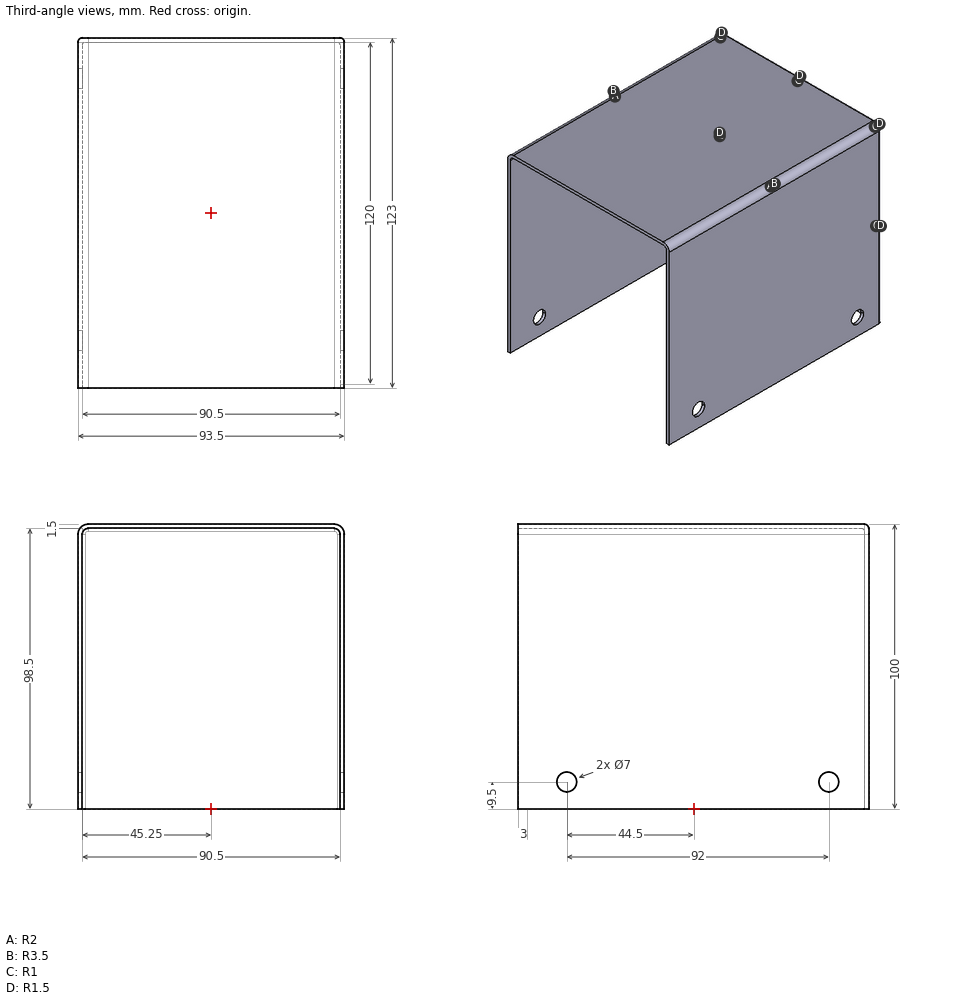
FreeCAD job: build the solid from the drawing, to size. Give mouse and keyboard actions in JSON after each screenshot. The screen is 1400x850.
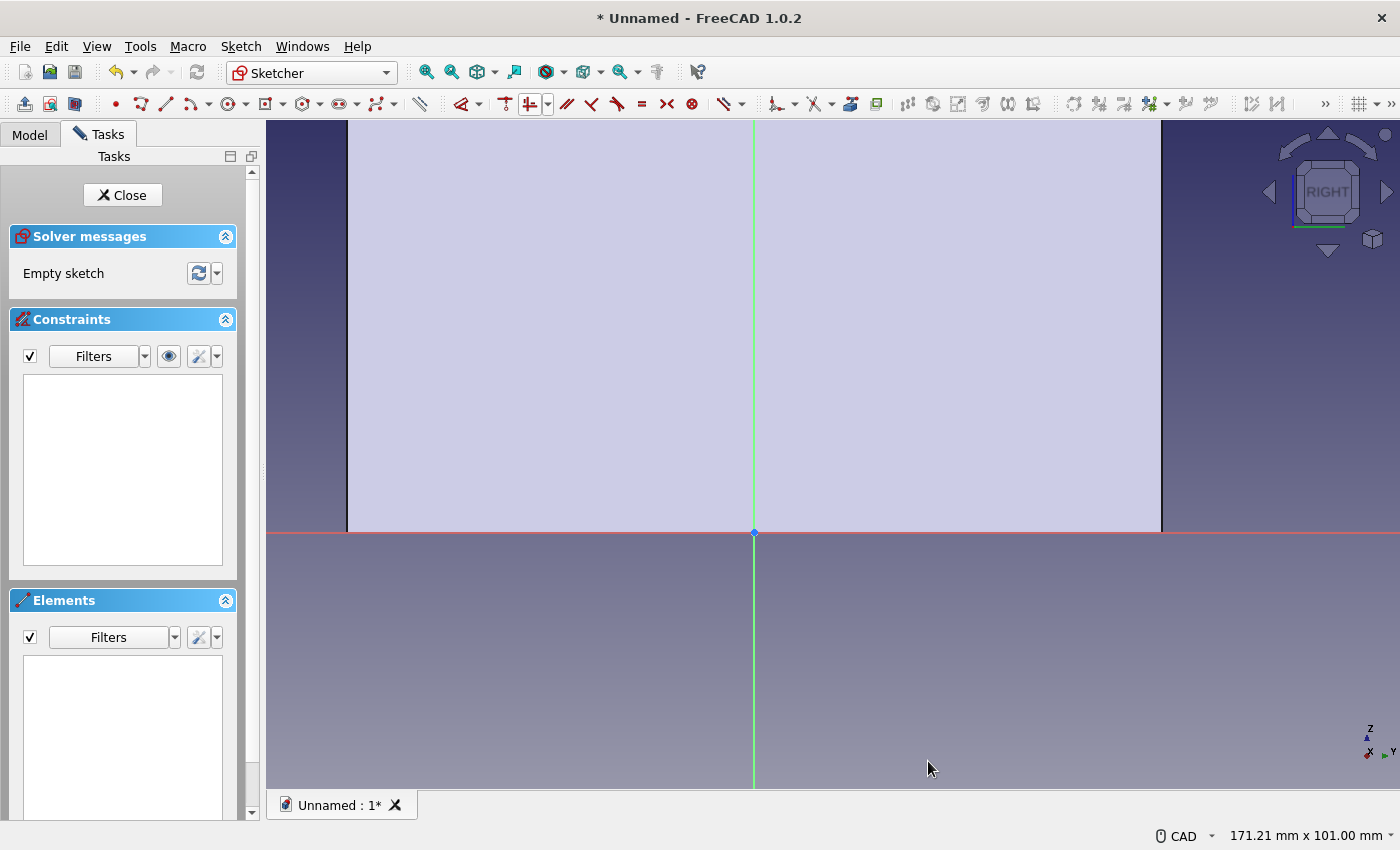
{"action": "left_click", "coordinate": [228, 104]}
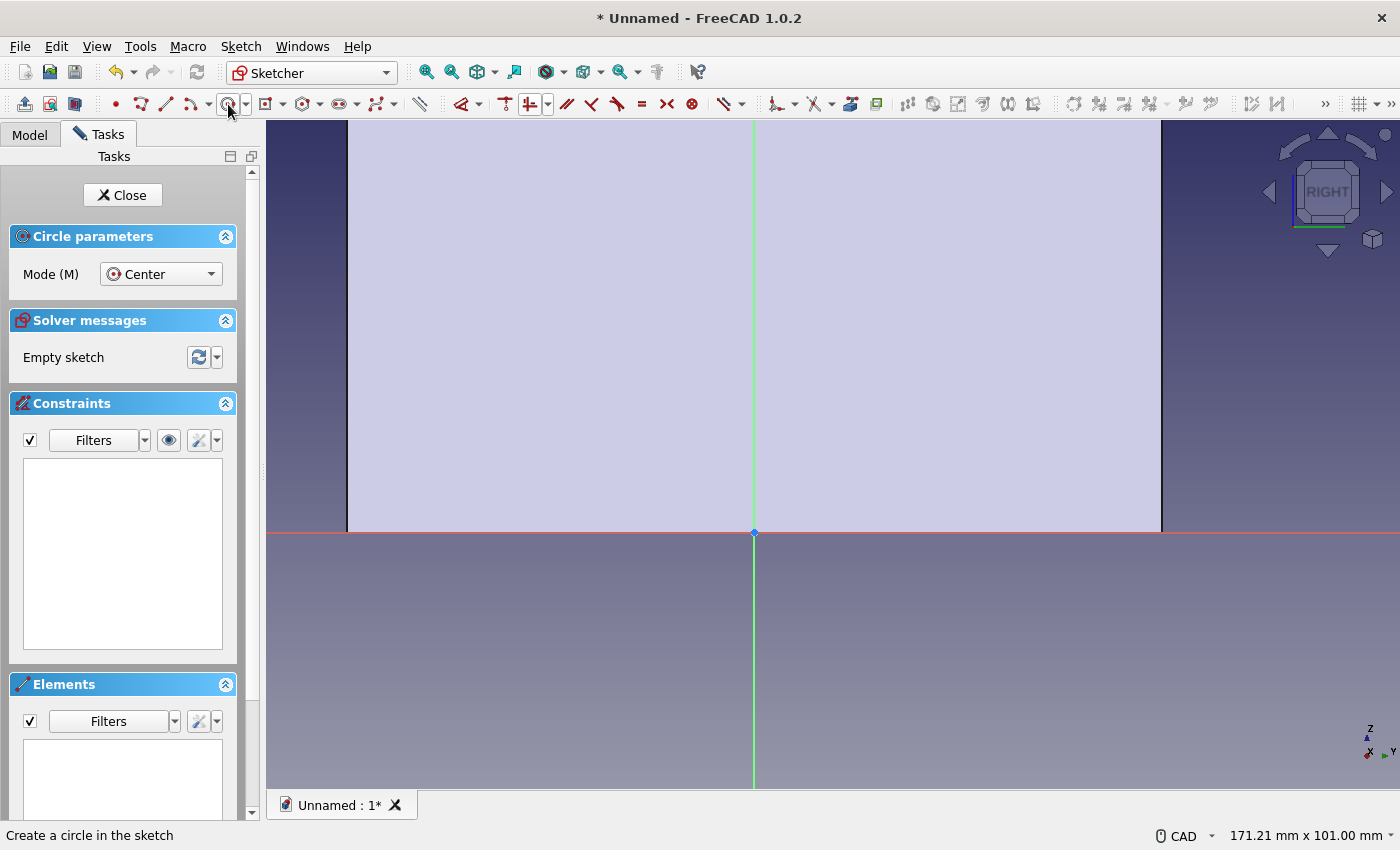
{"action": "left_click", "coordinate": [460, 470]}
{"action": "mouse_move", "coordinate": [476, 454]}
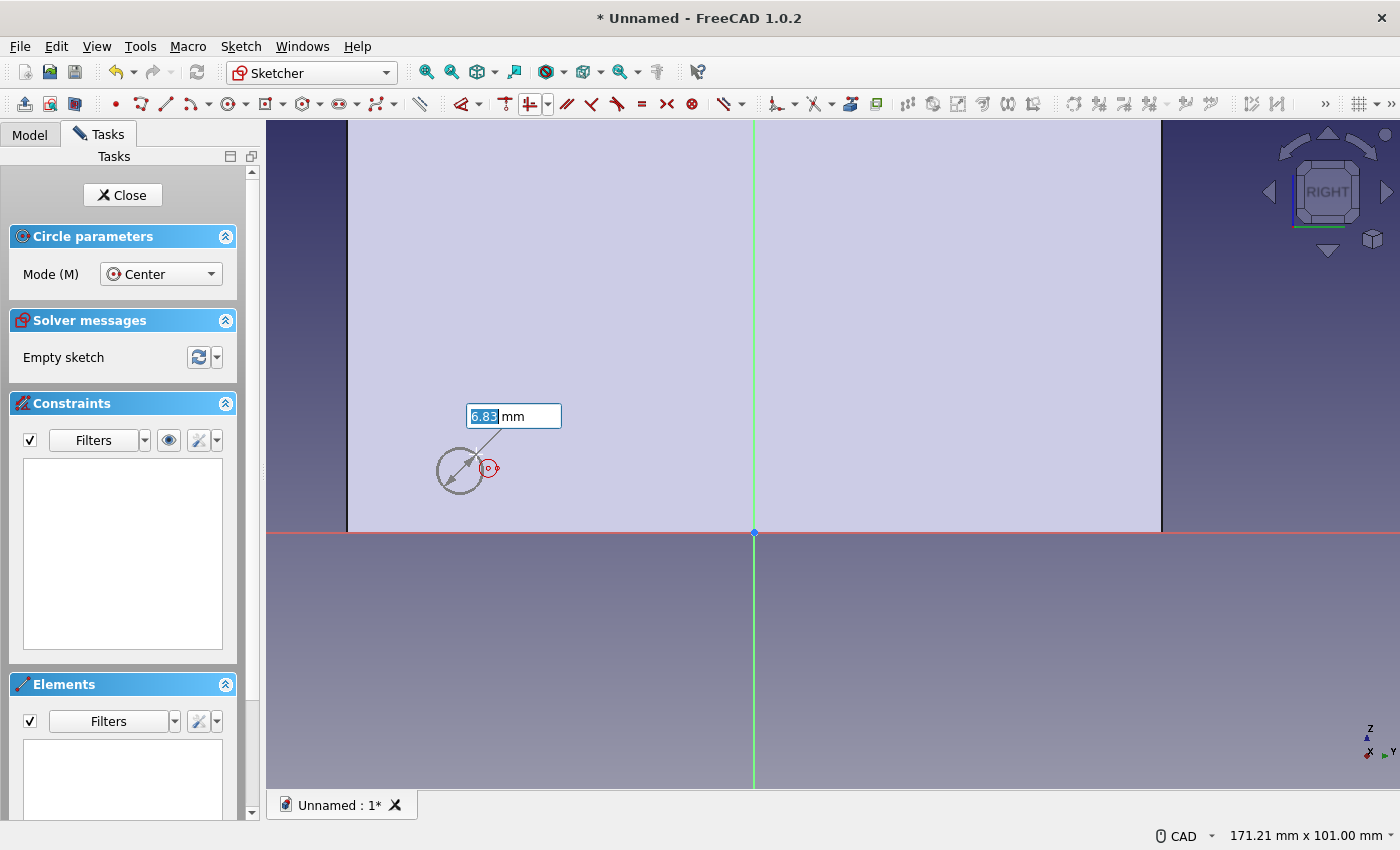
{"action": "type", "text": "7"}
{"action": "key", "text": "Return"}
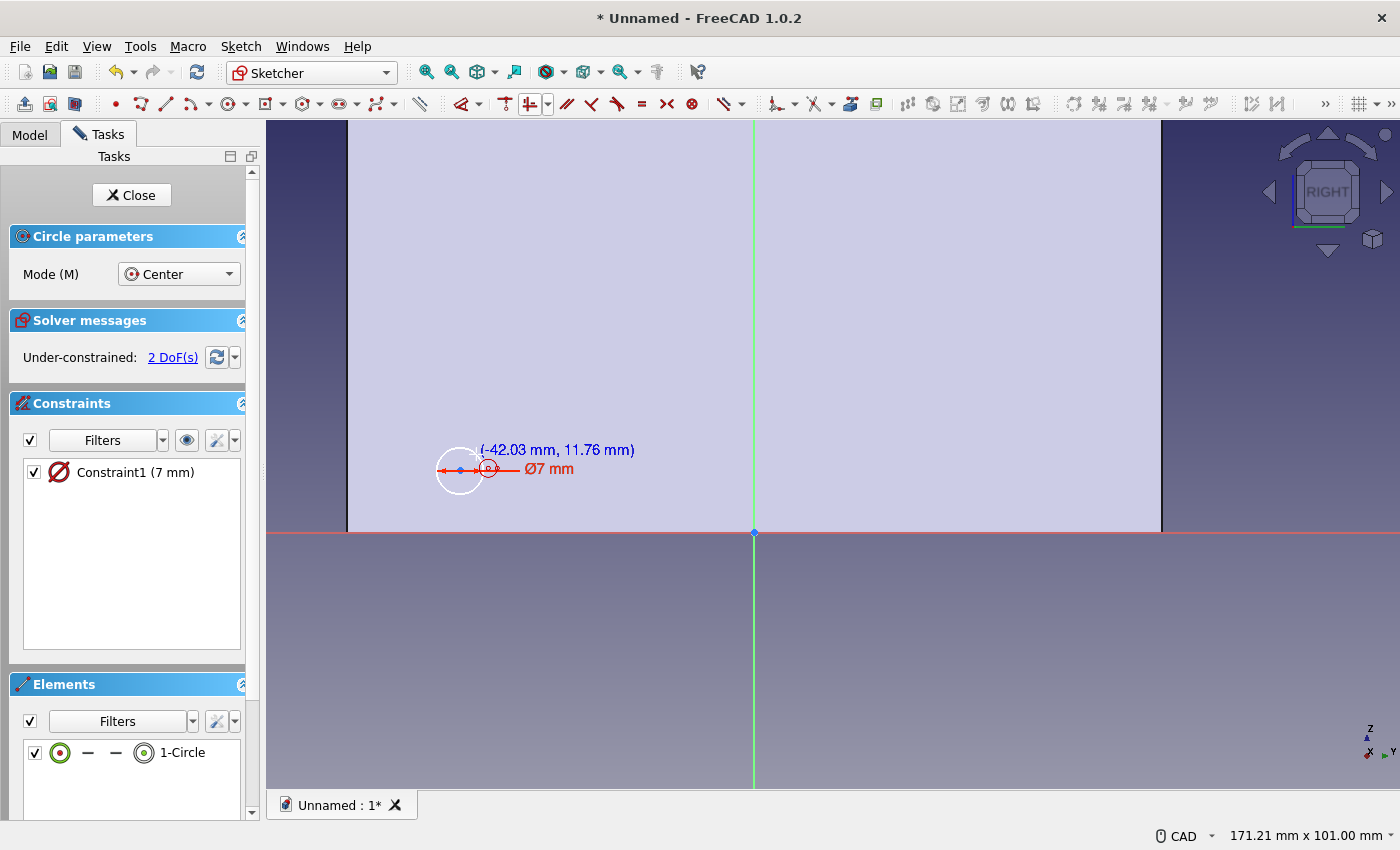
{"action": "left_click", "coordinate": [1069, 470]}
{"action": "mouse_move", "coordinate": [1085, 454]}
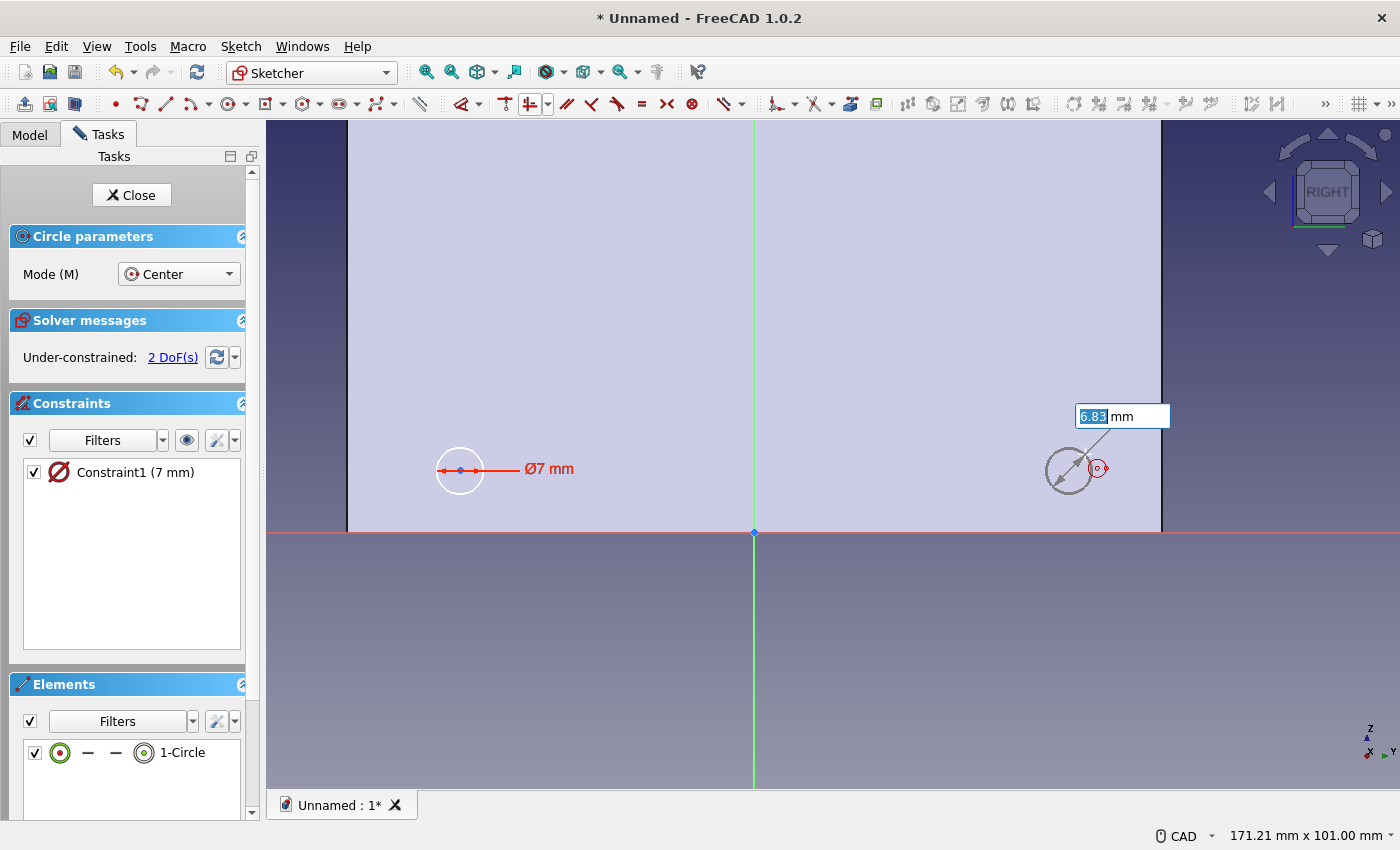
{"action": "type", "text": "7"}
{"action": "key", "text": "Return"}
{"action": "key", "text": "Escape"}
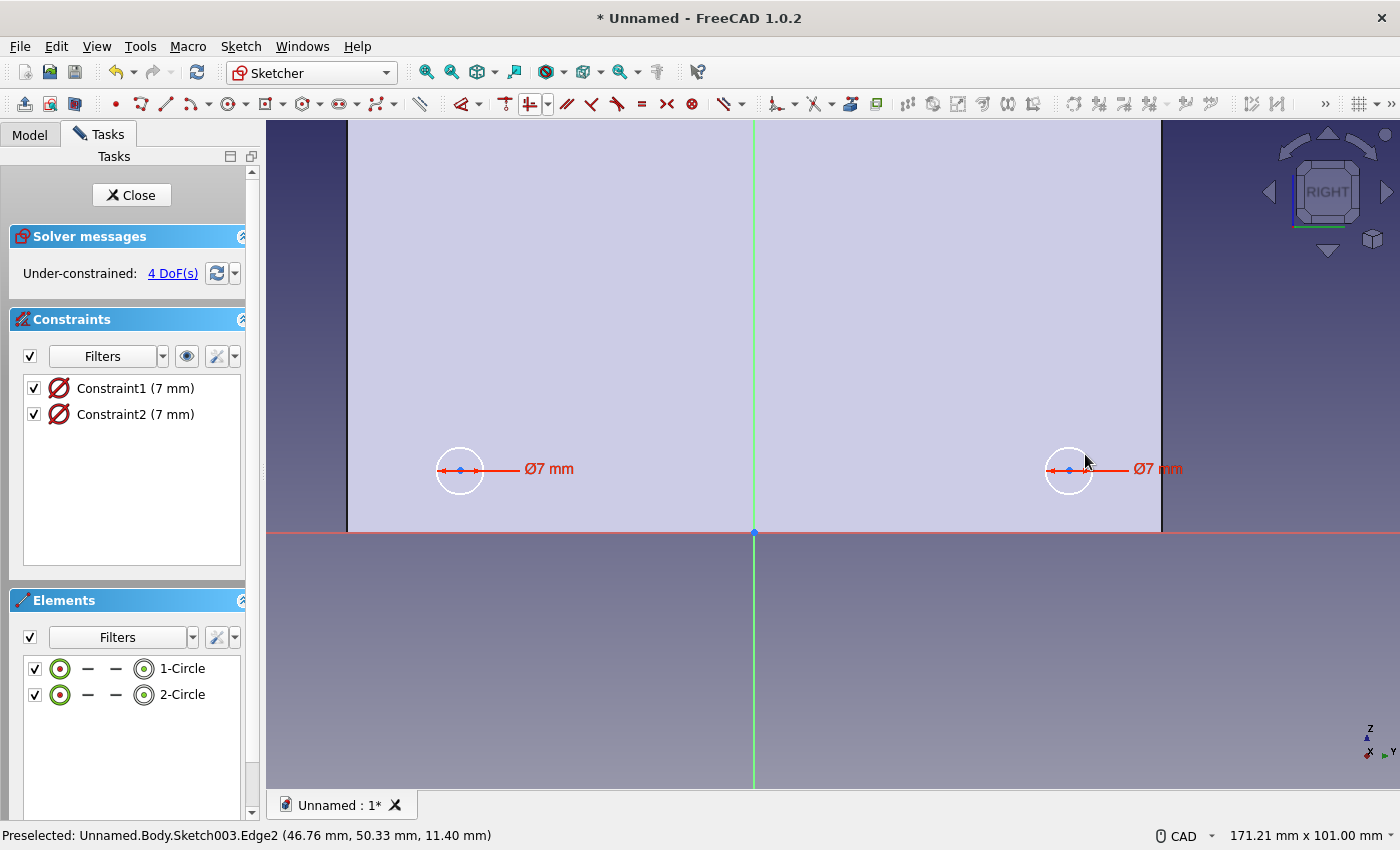
{"action": "left_click", "coordinate": [460, 471]}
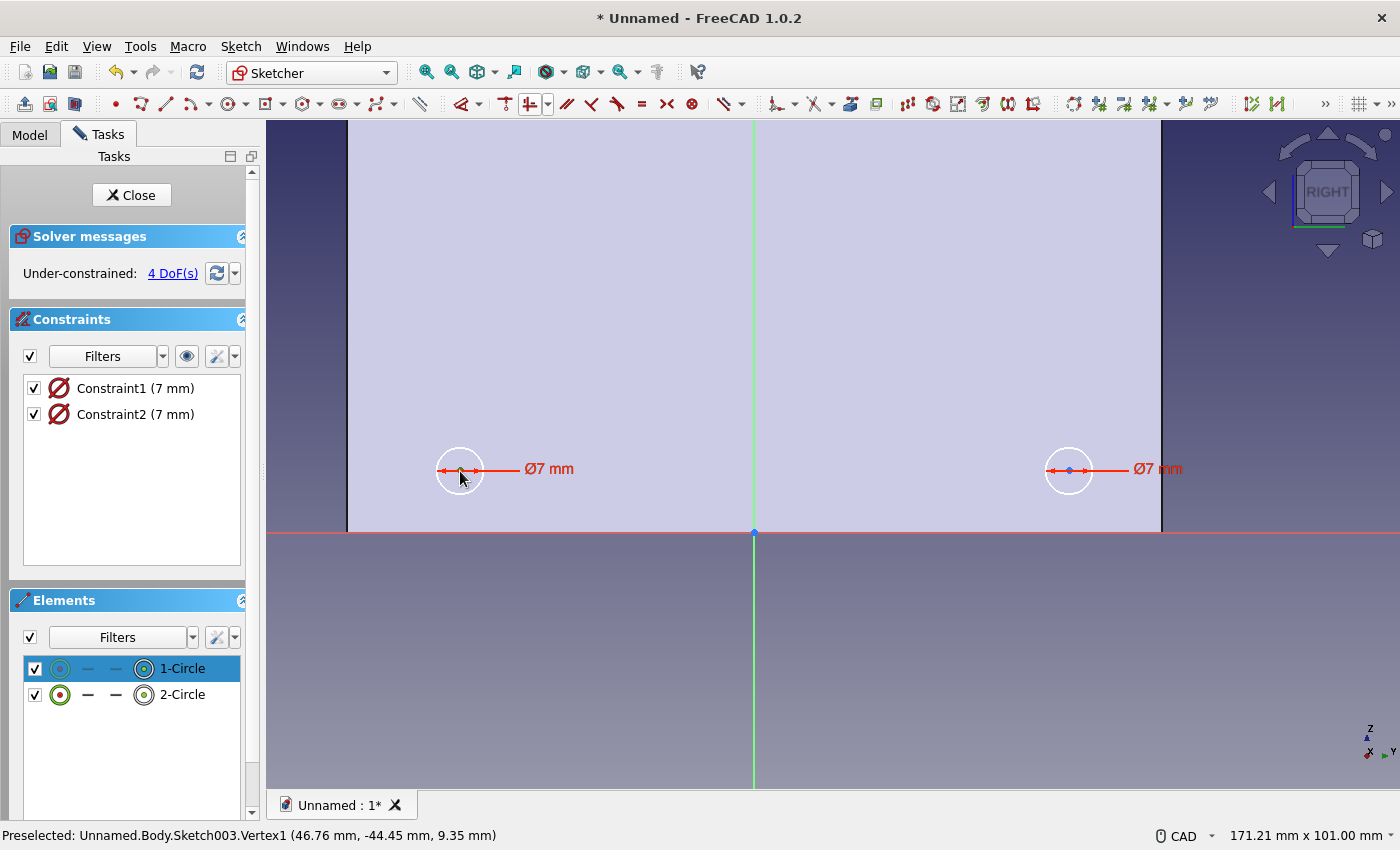
{"action": "left_click", "coordinate": [1069, 471]}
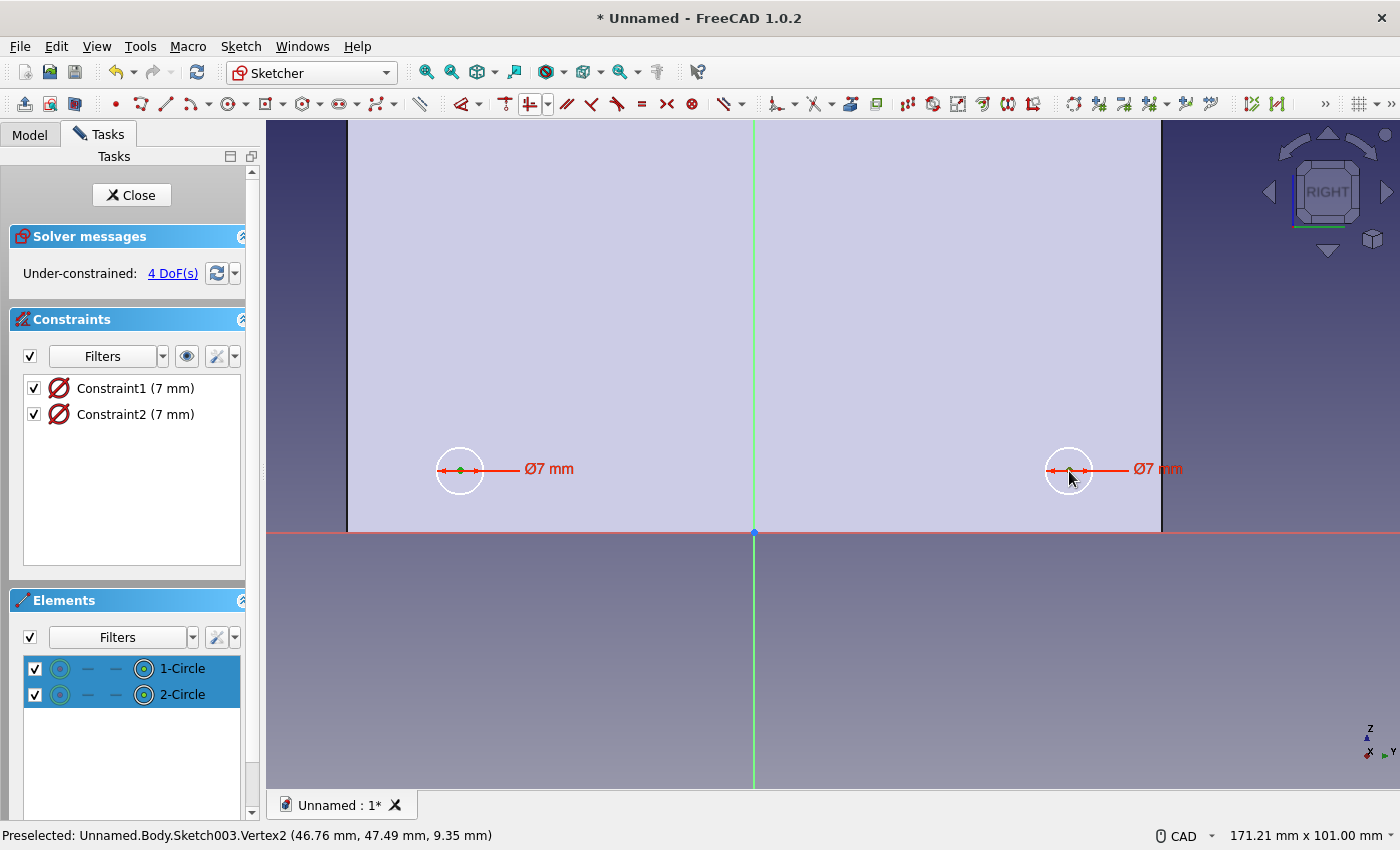
{"action": "left_click", "coordinate": [548, 104]}